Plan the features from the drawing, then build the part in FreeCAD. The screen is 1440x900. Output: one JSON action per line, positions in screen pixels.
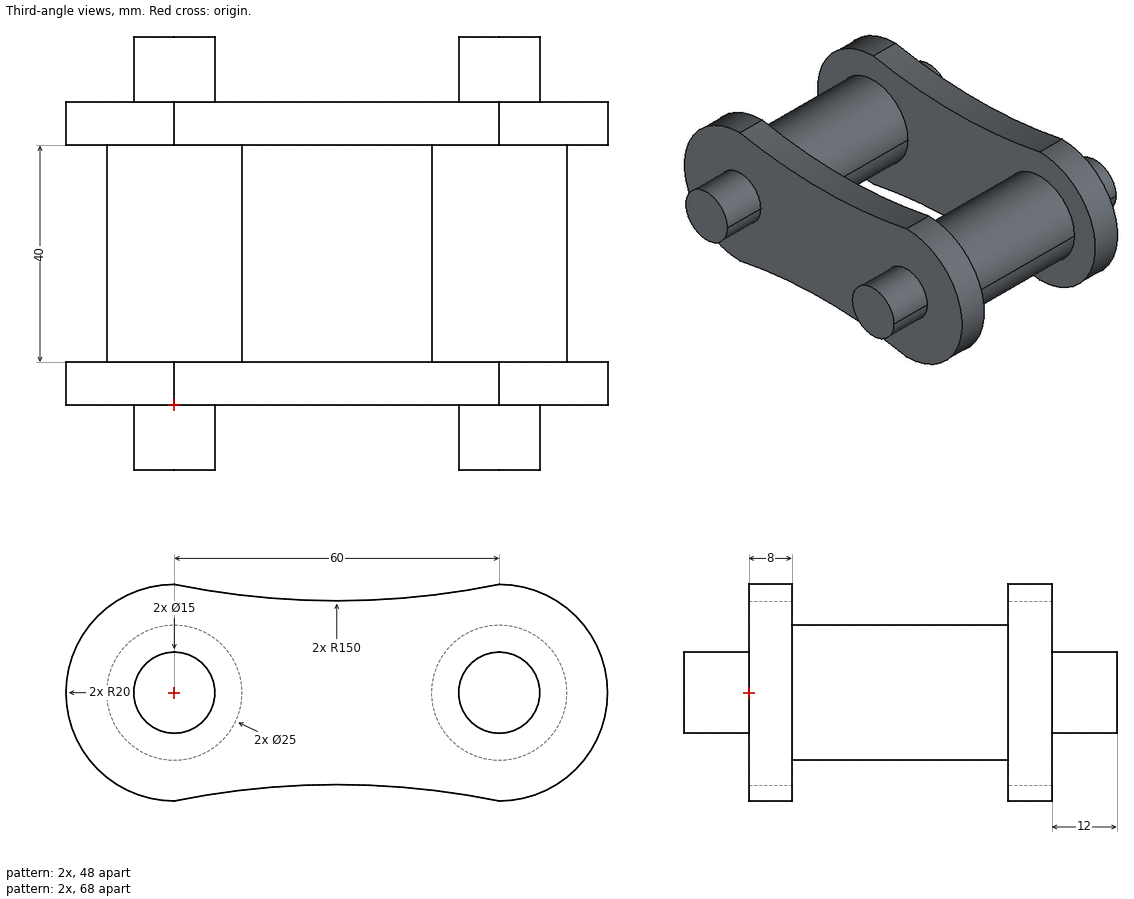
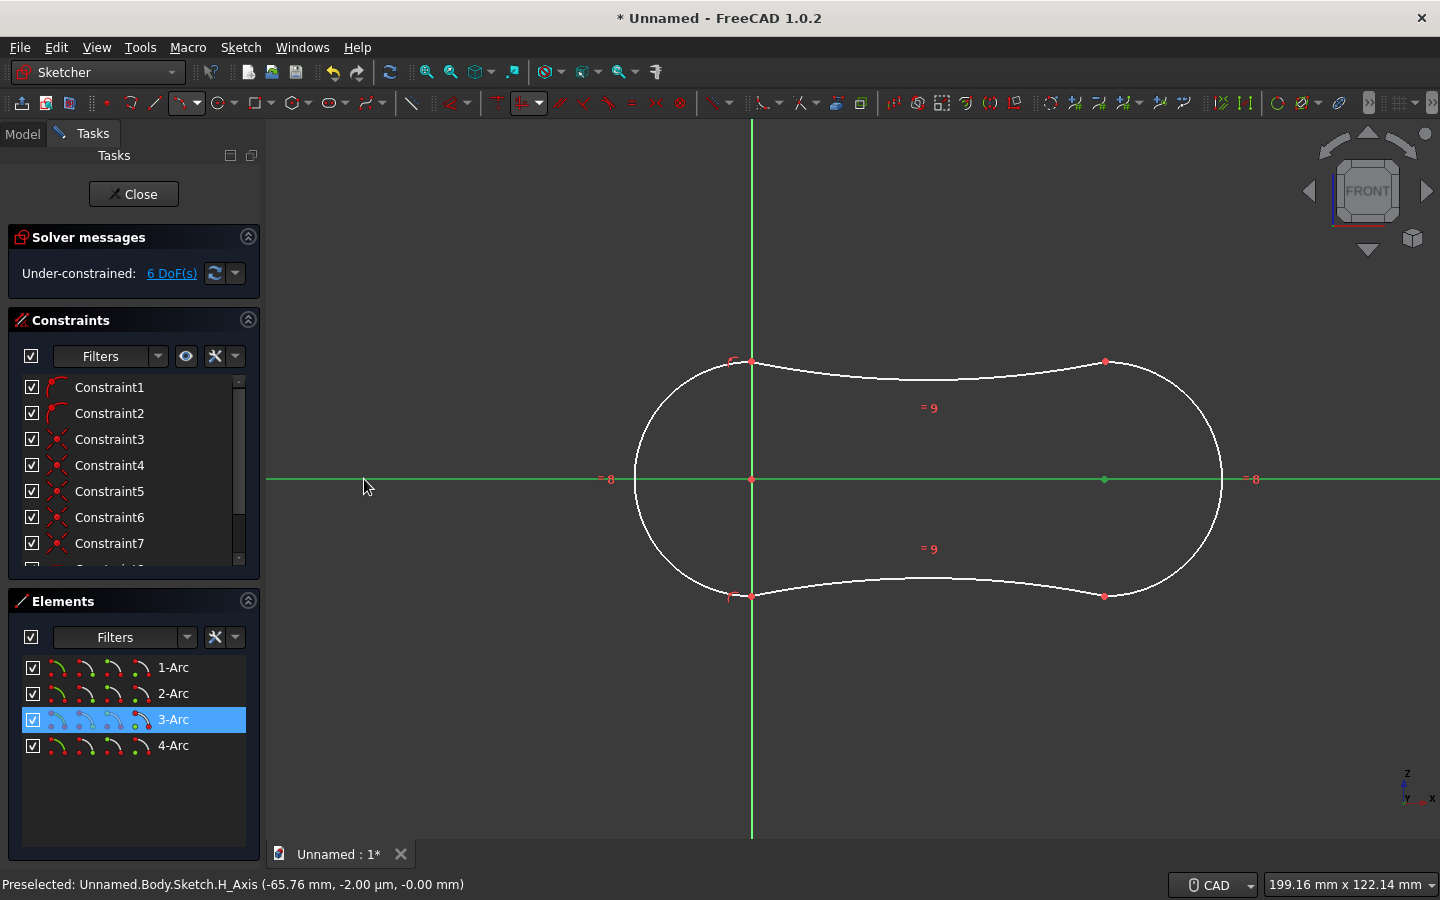
{"action": "left_click", "coordinate": [498, 104]}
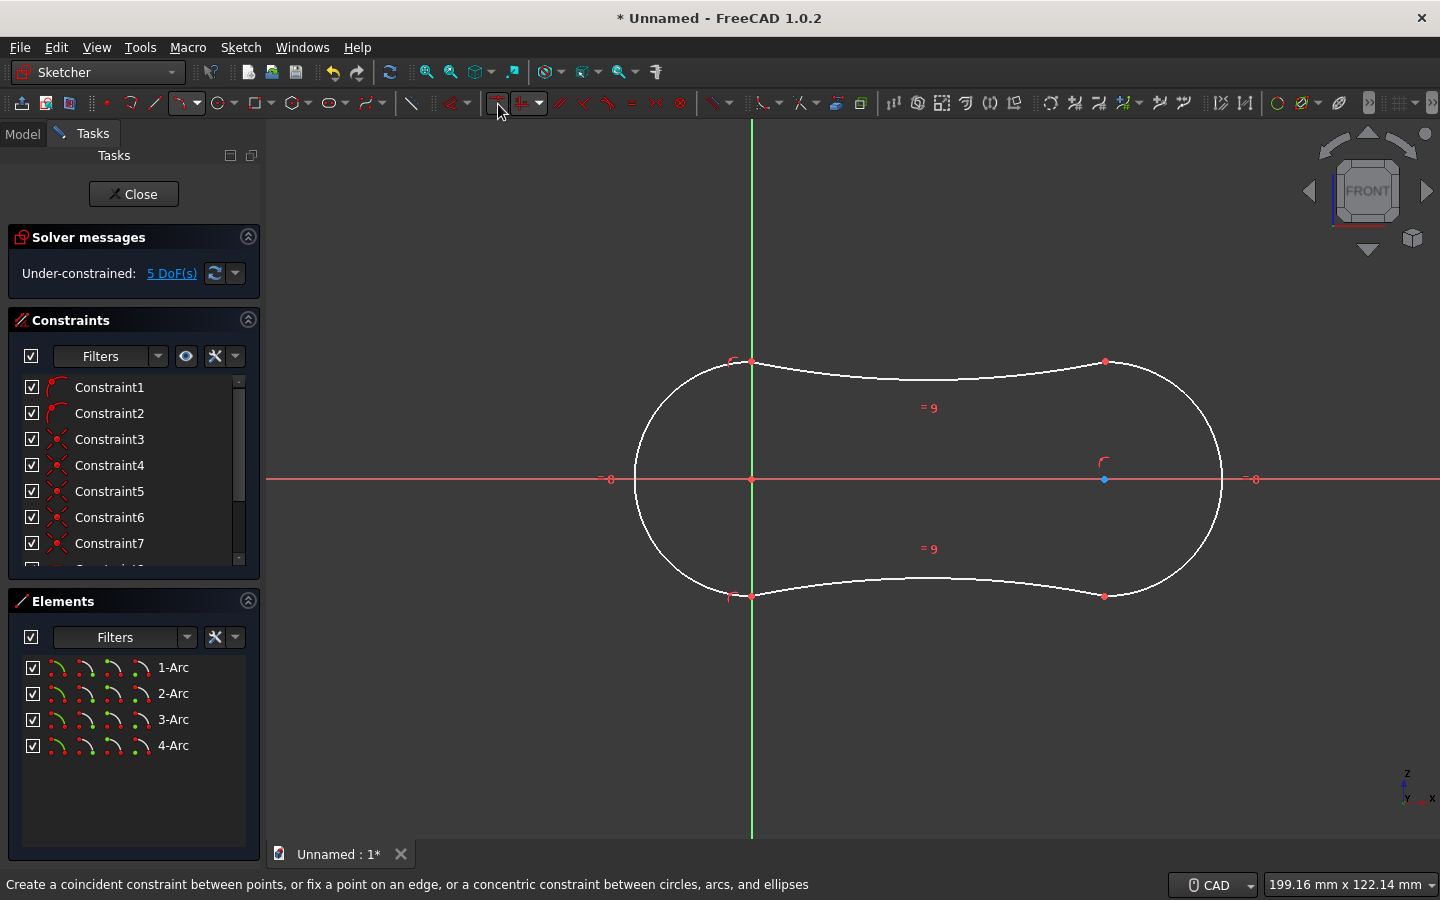
{"action": "left_click", "coordinate": [450, 104]}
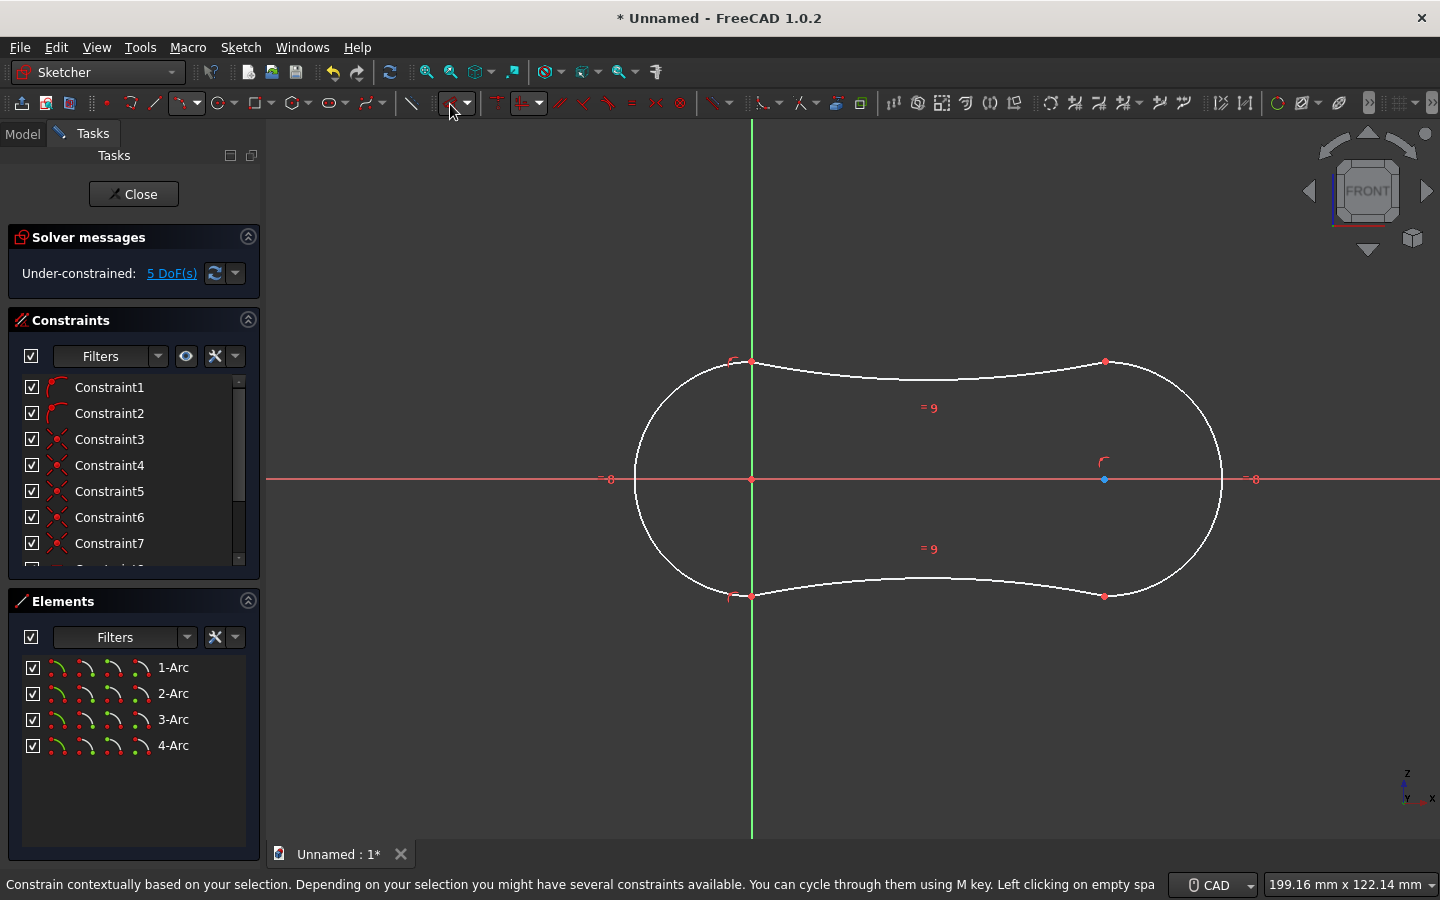
{"action": "left_click", "coordinate": [657, 410]}
{"action": "left_click", "coordinate": [631, 391]}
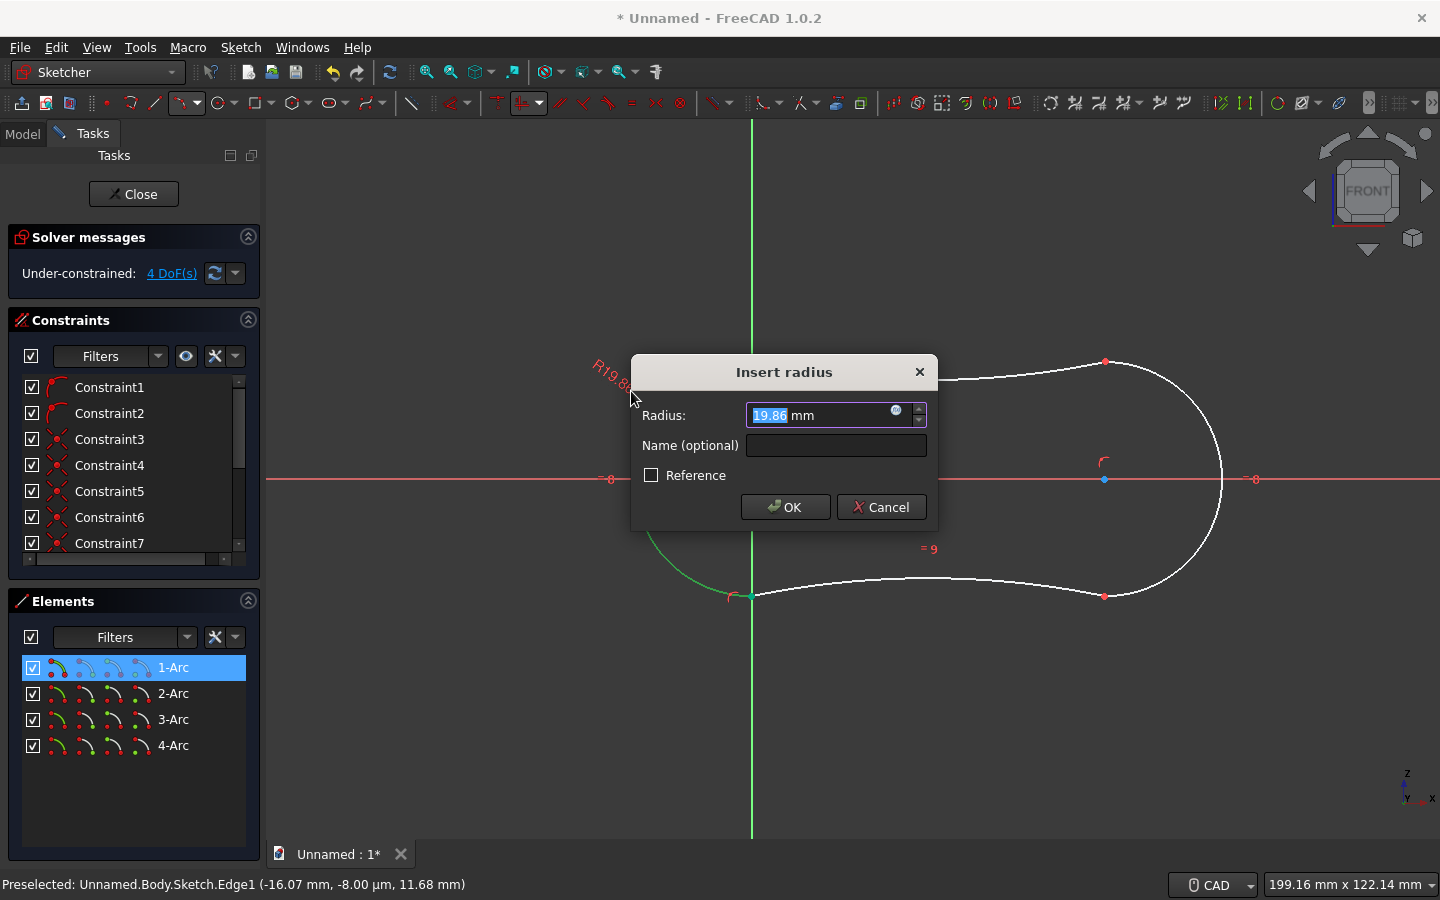
{"action": "type", "text": "20"}
{"action": "key", "text": "Return"}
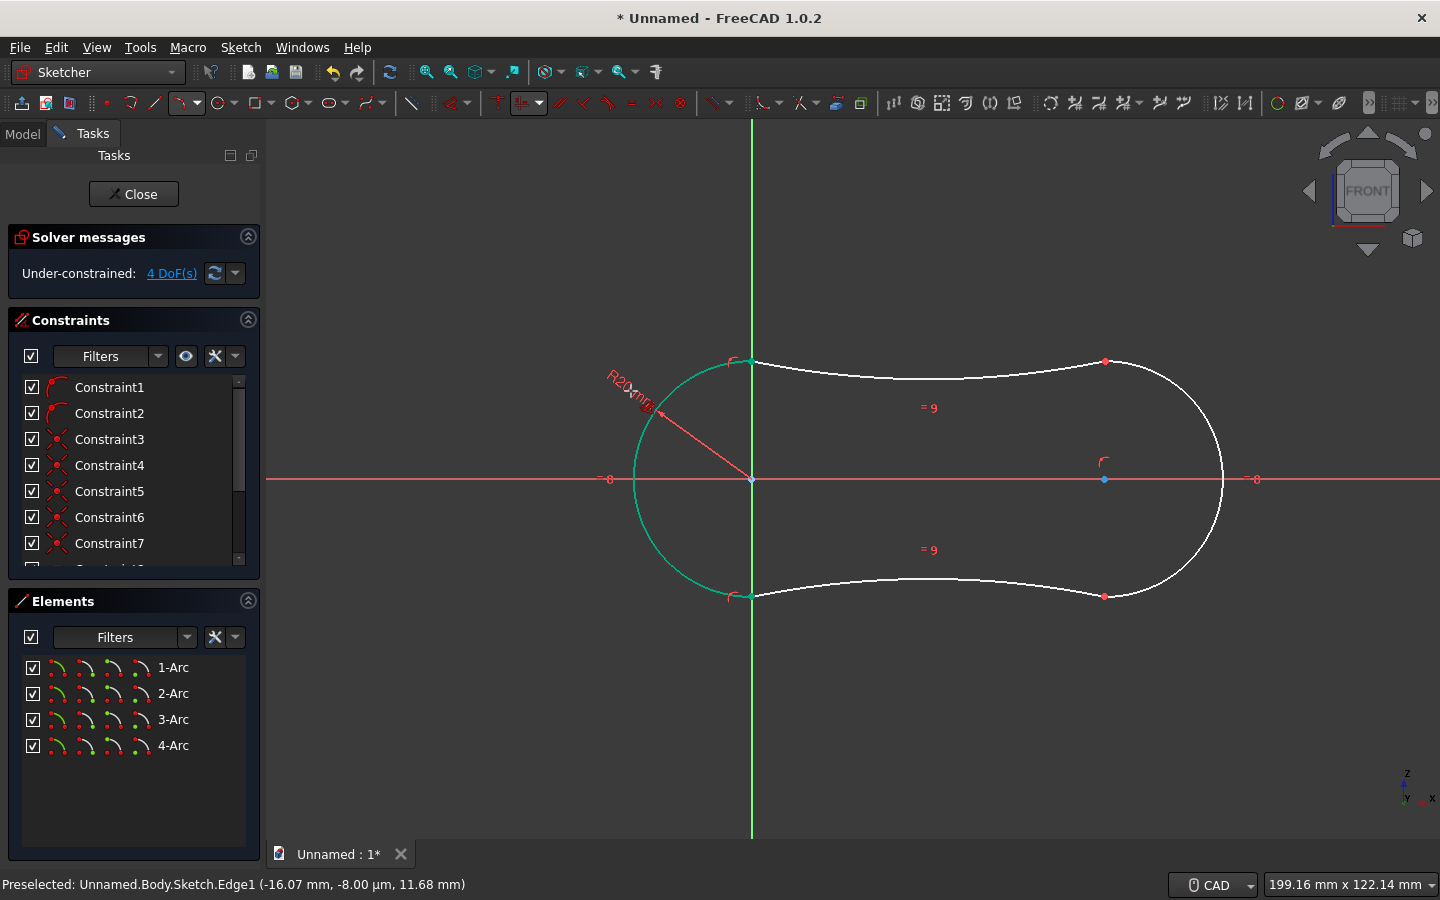
{"action": "left_click", "coordinate": [857, 376]}
{"action": "left_click", "coordinate": [854, 408]}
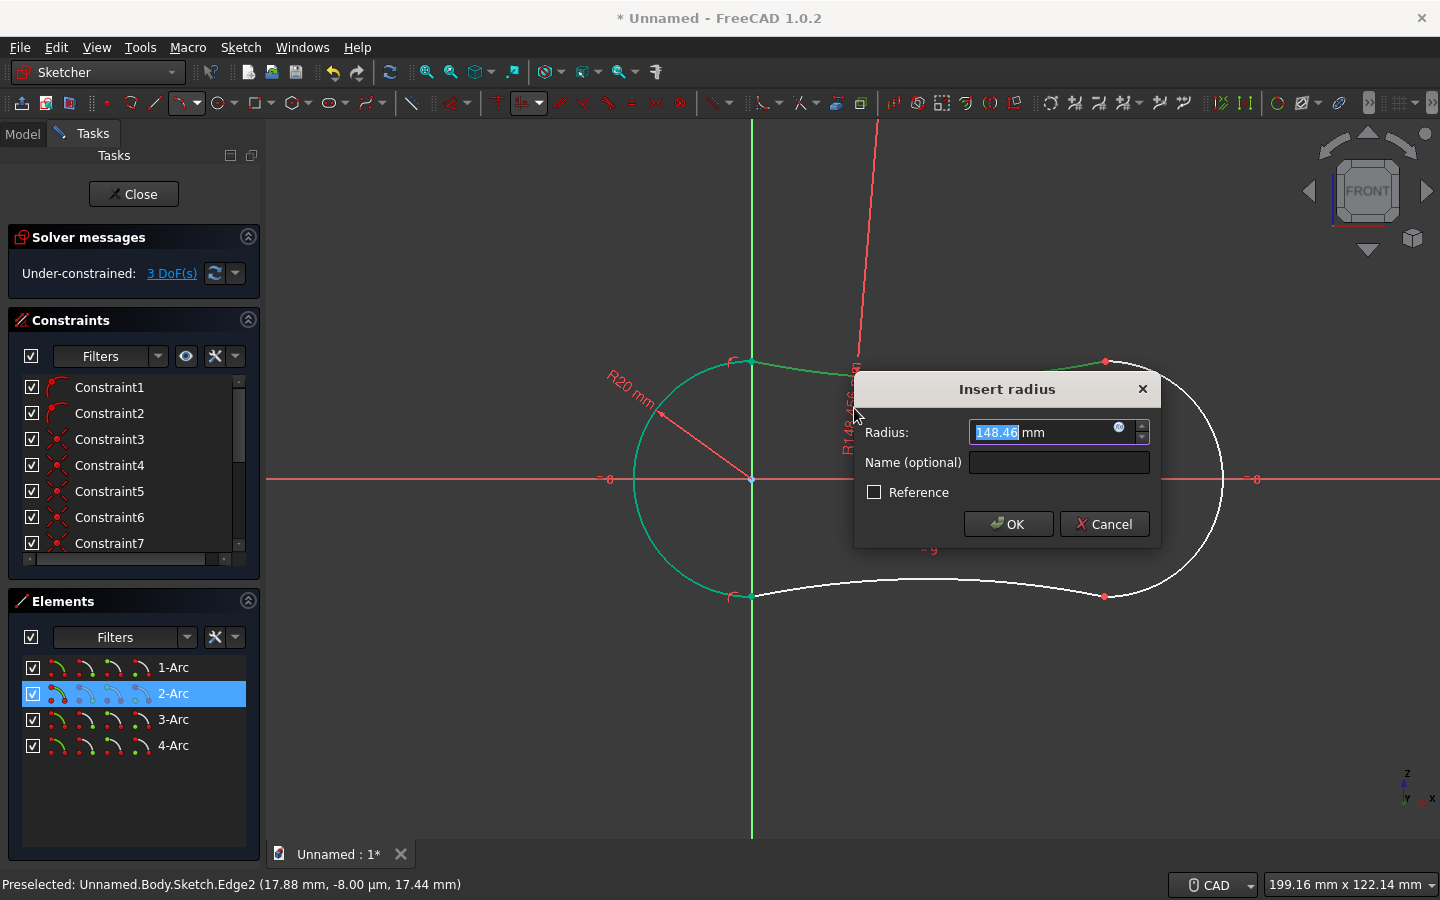
{"action": "type", "text": "150"}
{"action": "key", "text": "Return"}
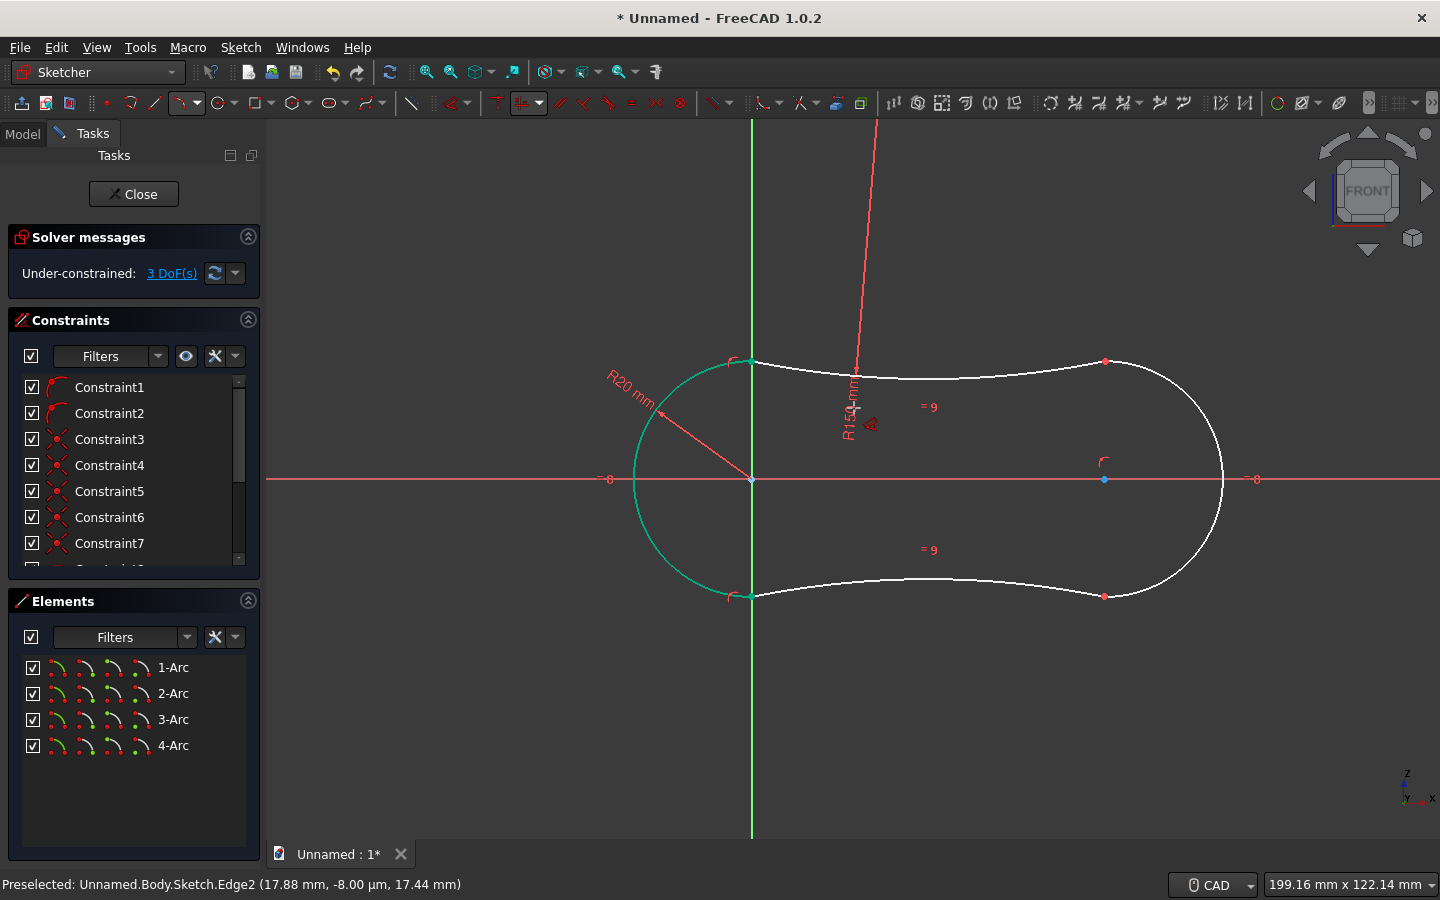
{"action": "left_click", "coordinate": [1105, 361]}
{"action": "left_click", "coordinate": [928, 327]}